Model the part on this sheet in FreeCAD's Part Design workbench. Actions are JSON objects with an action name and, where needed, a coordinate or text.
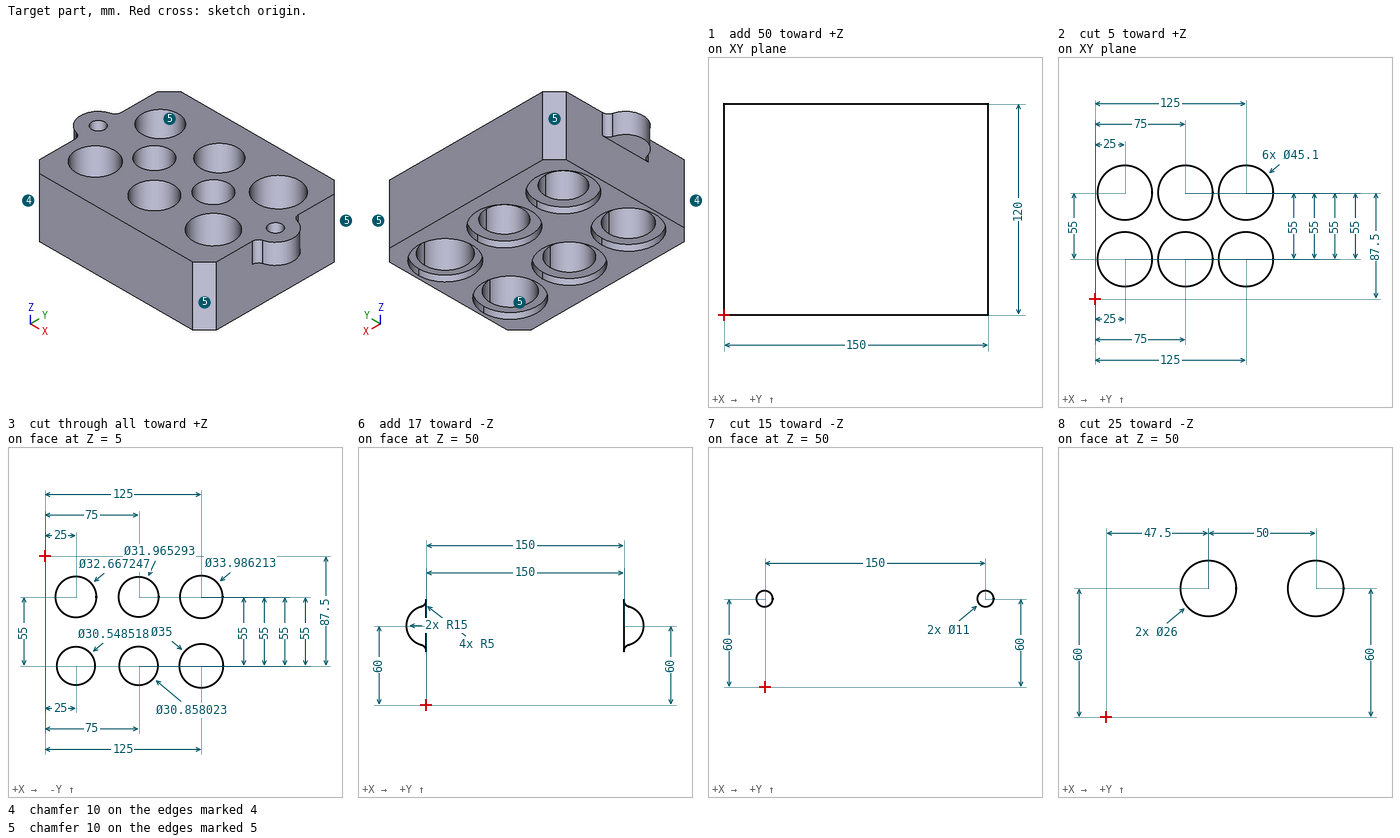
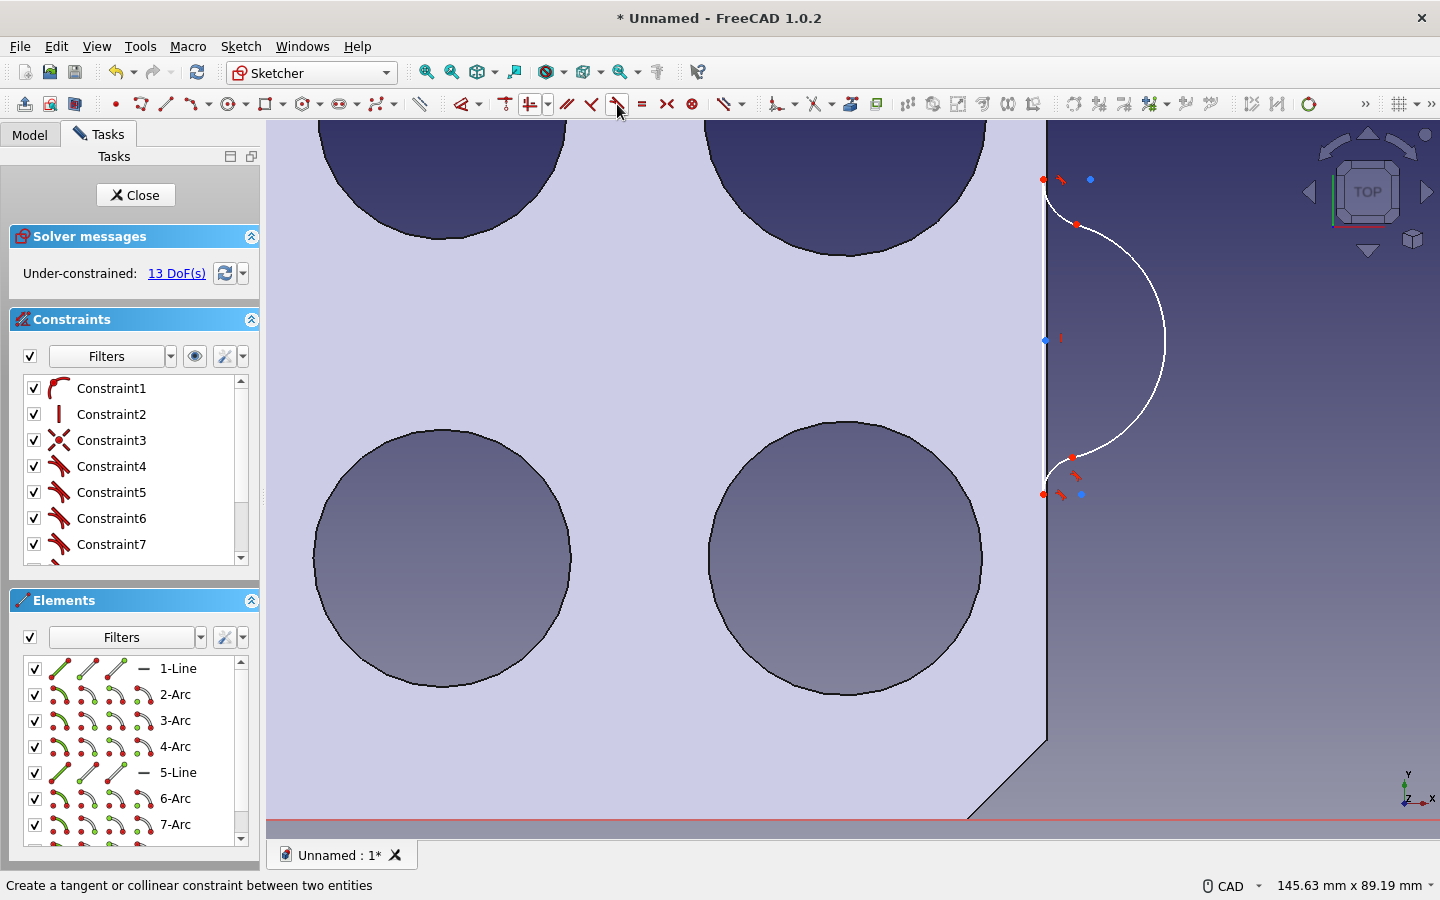
{"action": "left_click", "coordinate": [1148, 403]}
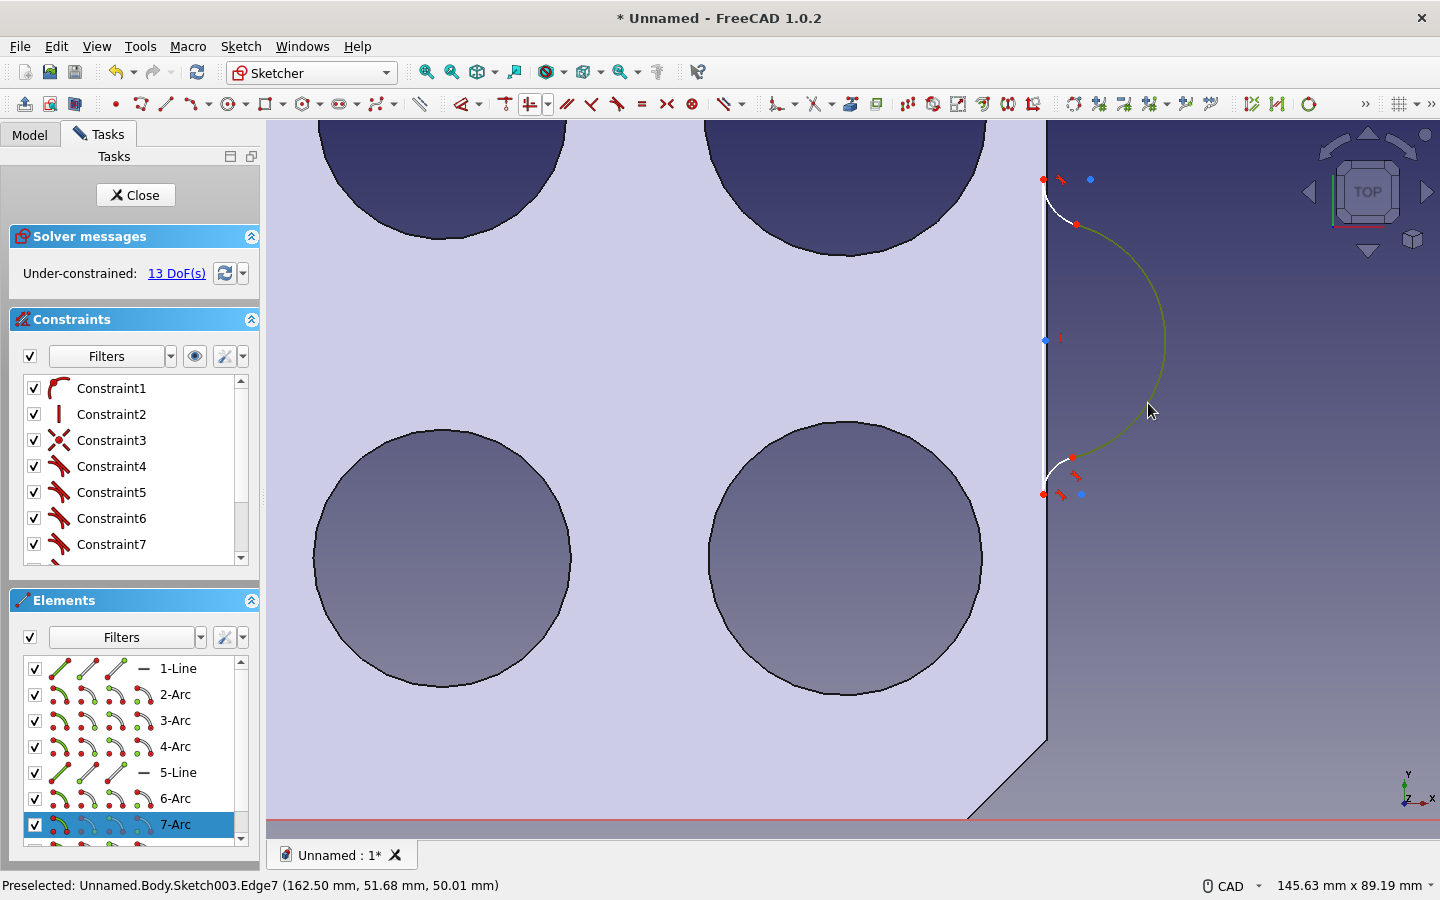
{"action": "left_click", "coordinate": [1061, 216]}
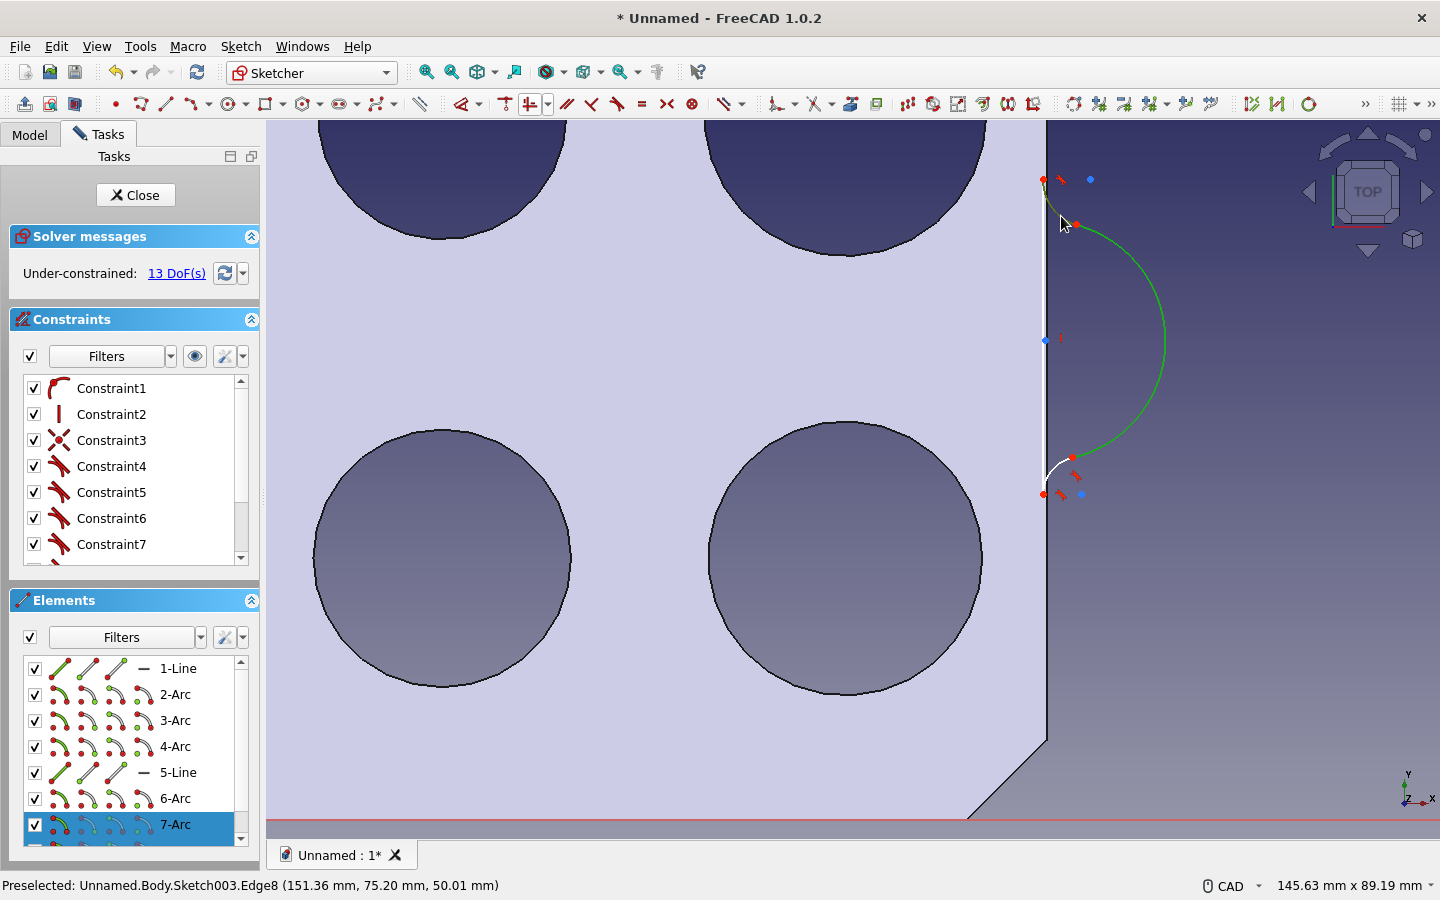
{"action": "left_click", "coordinate": [617, 104]}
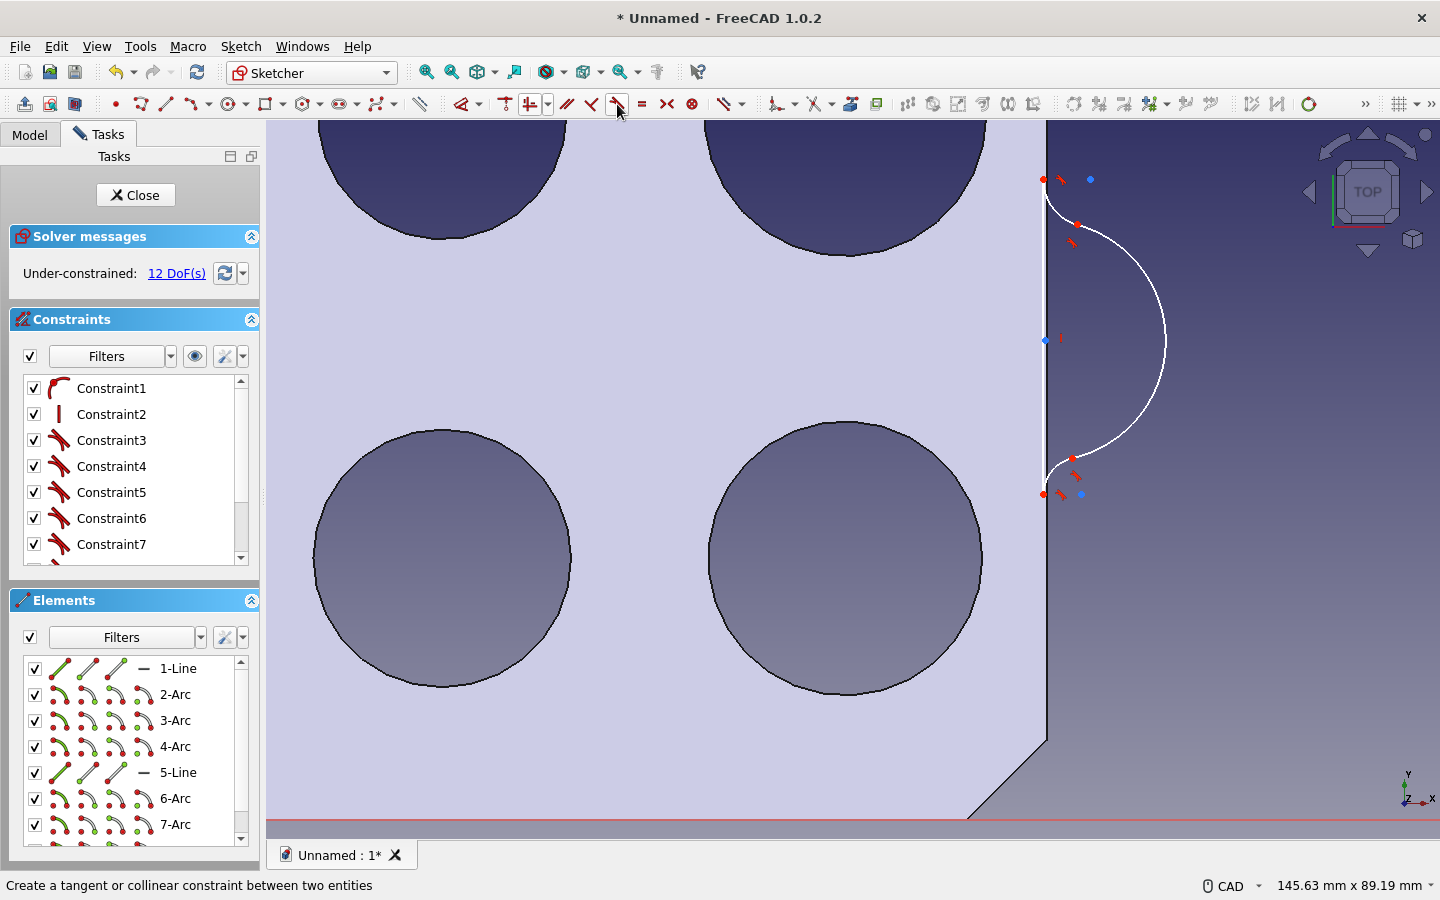
{"action": "scroll", "coordinate": [1064, 462], "scroll_direction": "down", "scroll_amount": 4}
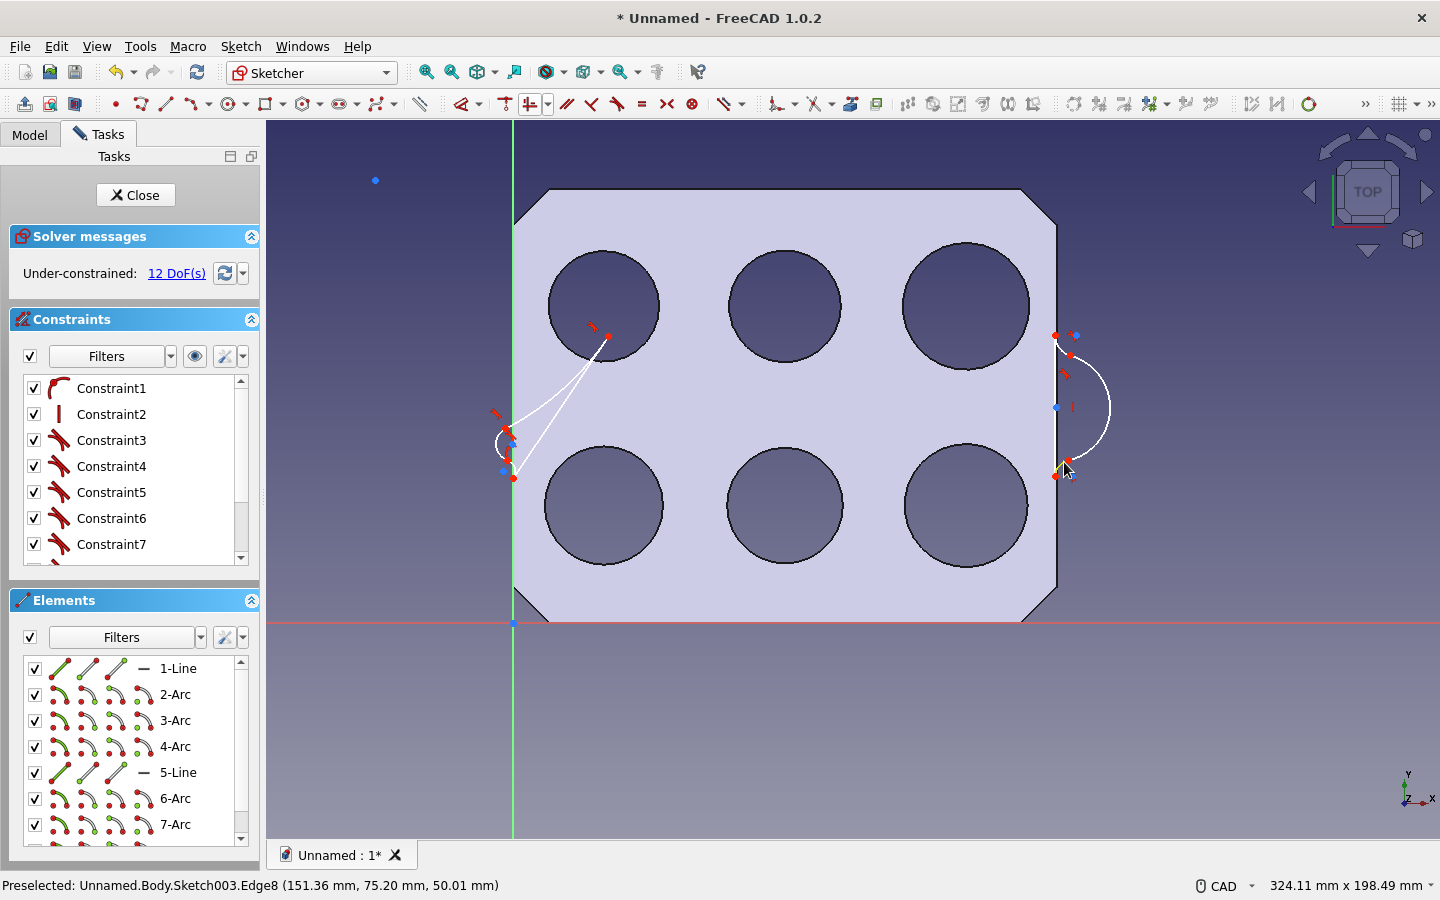
{"action": "left_click", "coordinate": [542, 436]}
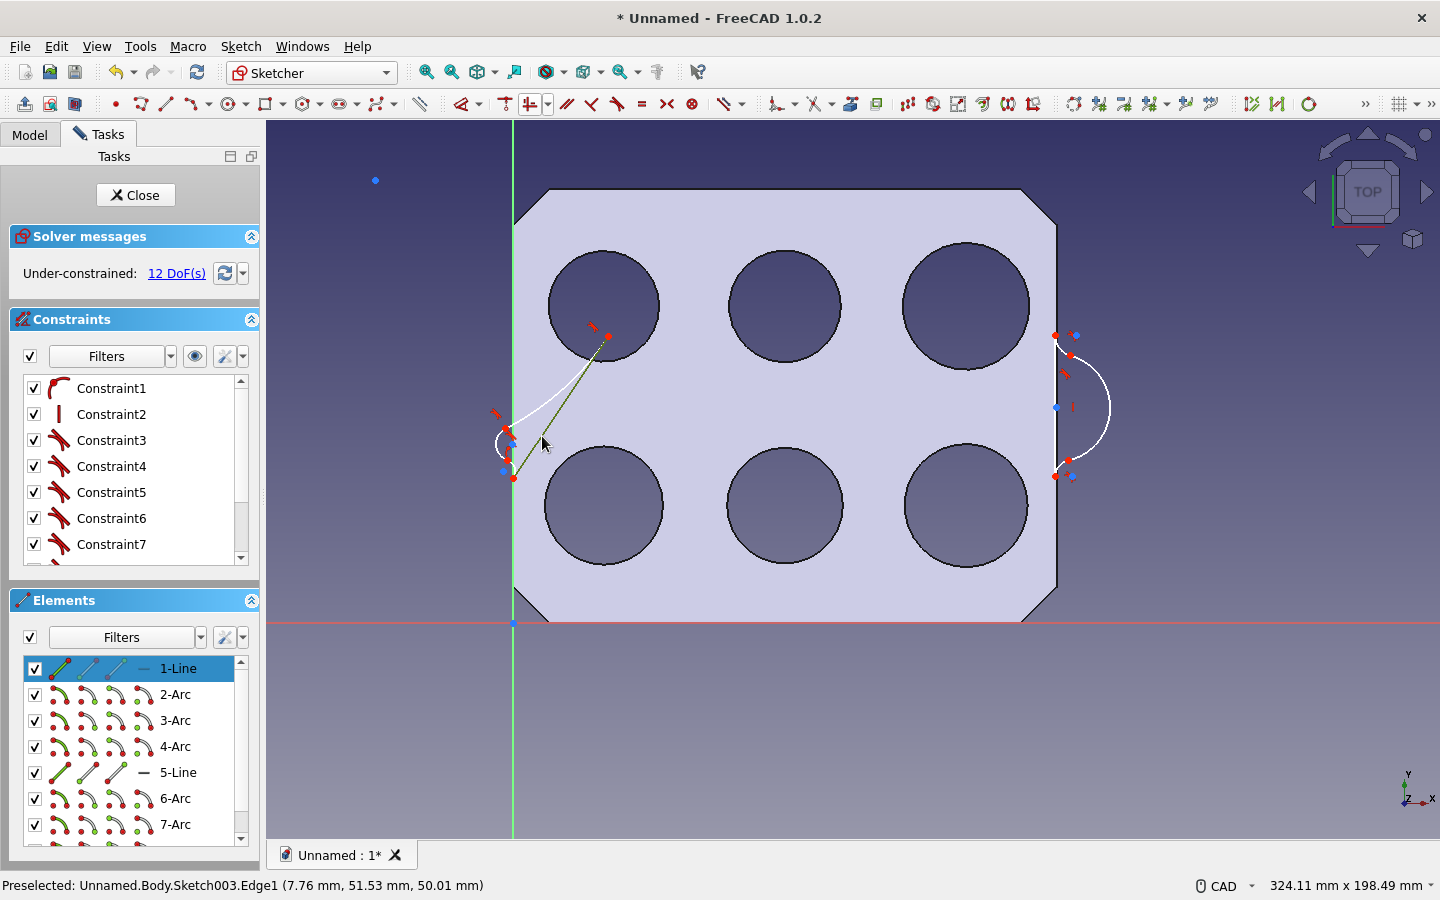
{"action": "key", "text": "v"}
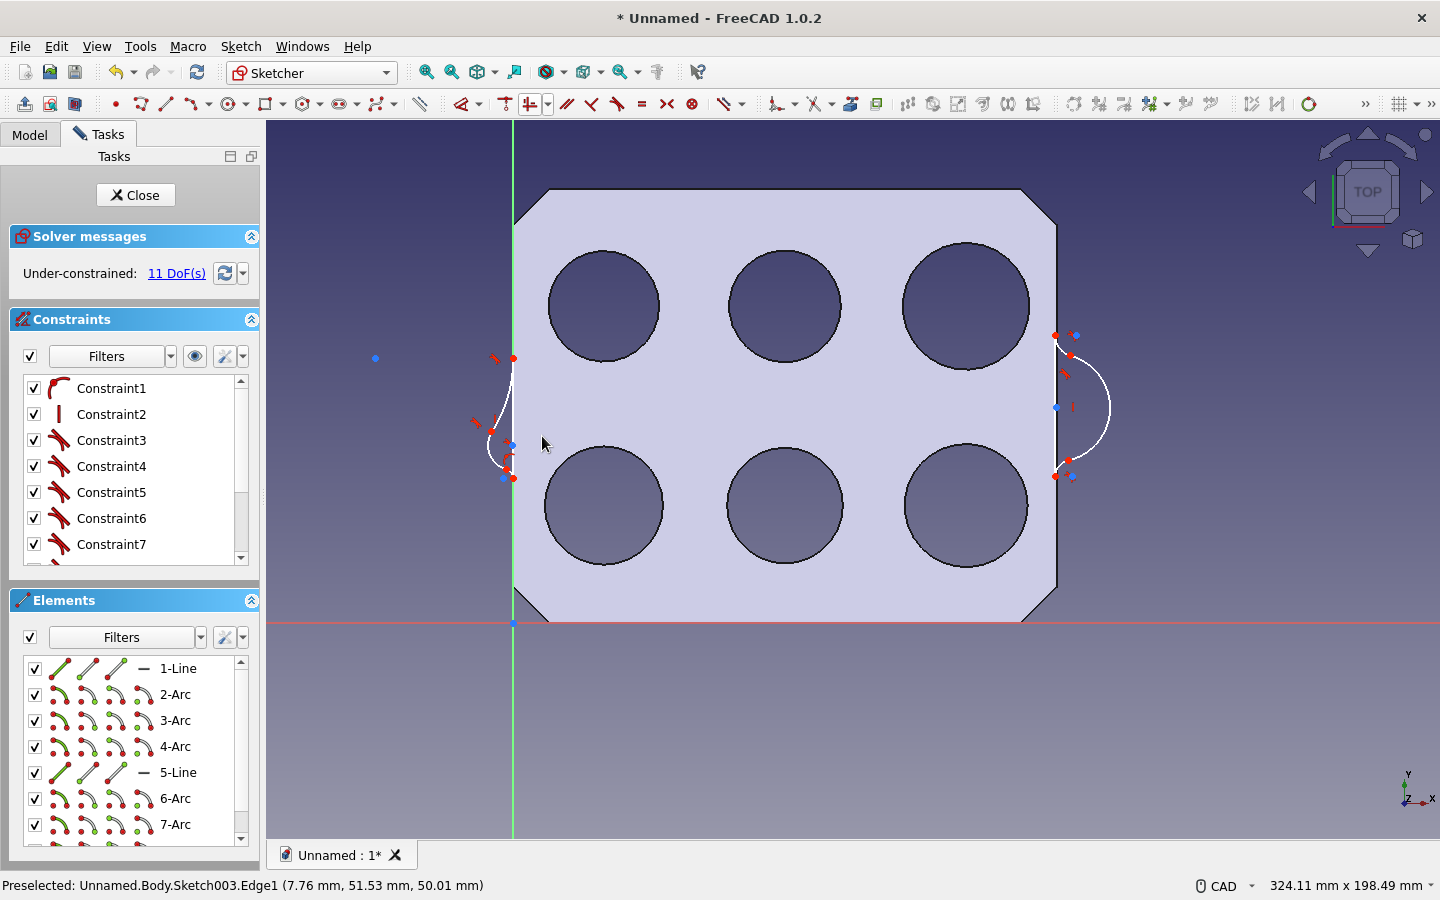
{"action": "scroll", "coordinate": [503, 411], "scroll_direction": "up", "scroll_amount": 2}